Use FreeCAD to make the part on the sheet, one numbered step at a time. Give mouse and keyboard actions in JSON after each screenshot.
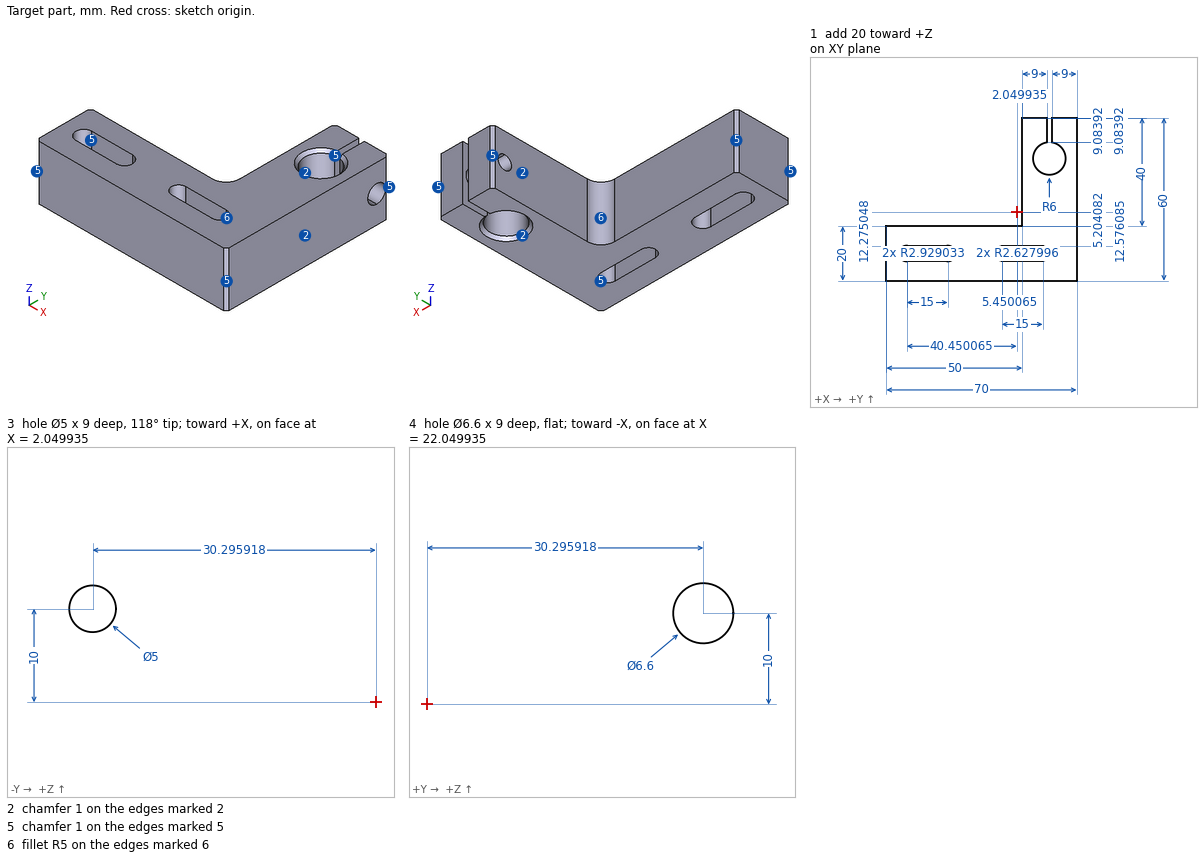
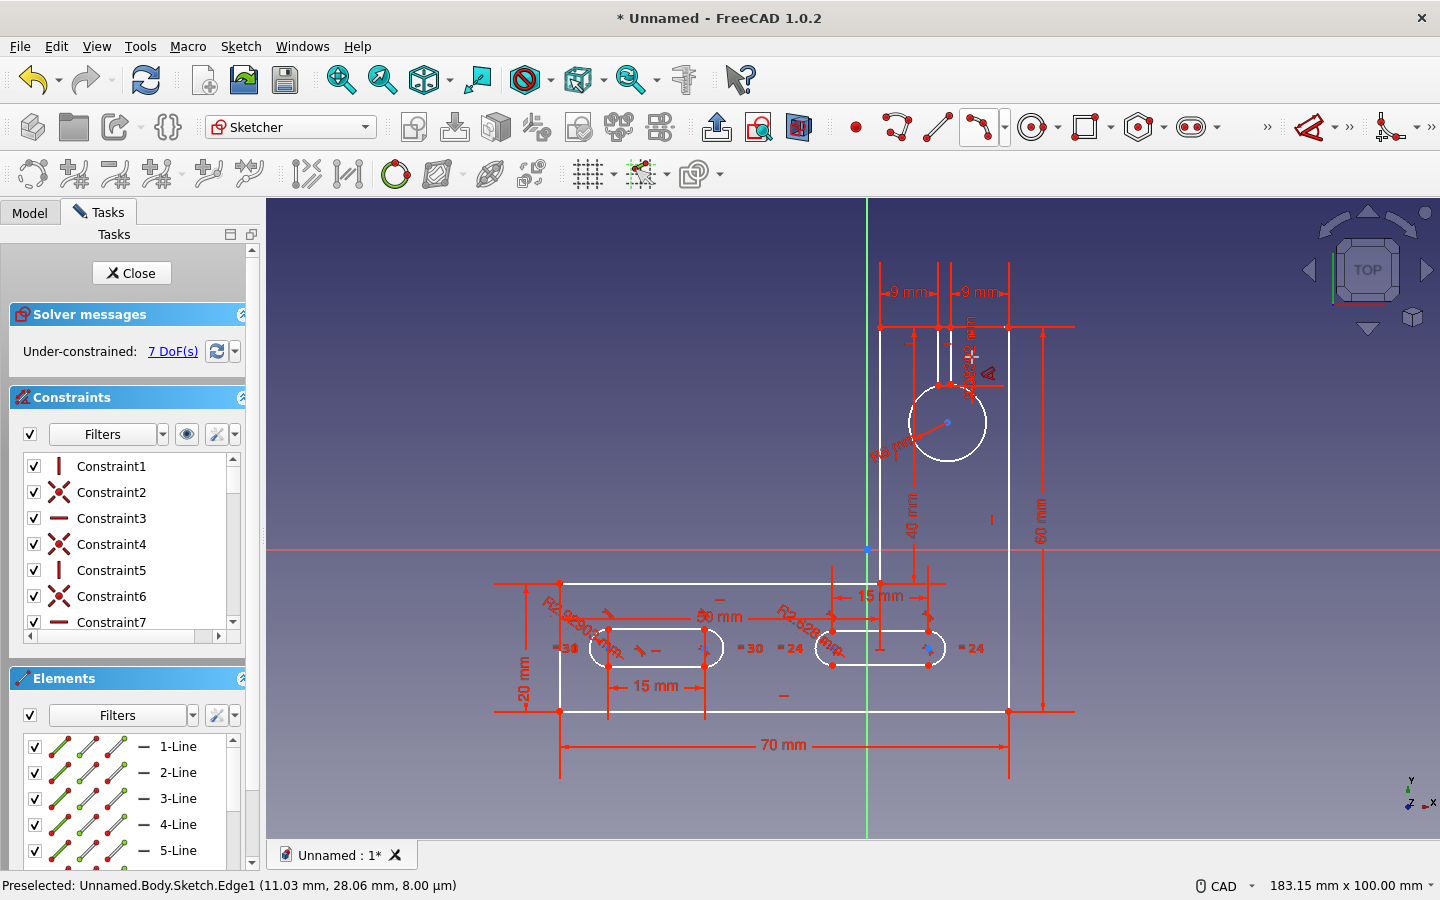
{"action": "left_click", "coordinate": [951, 345]}
{"action": "left_click", "coordinate": [1033, 336]}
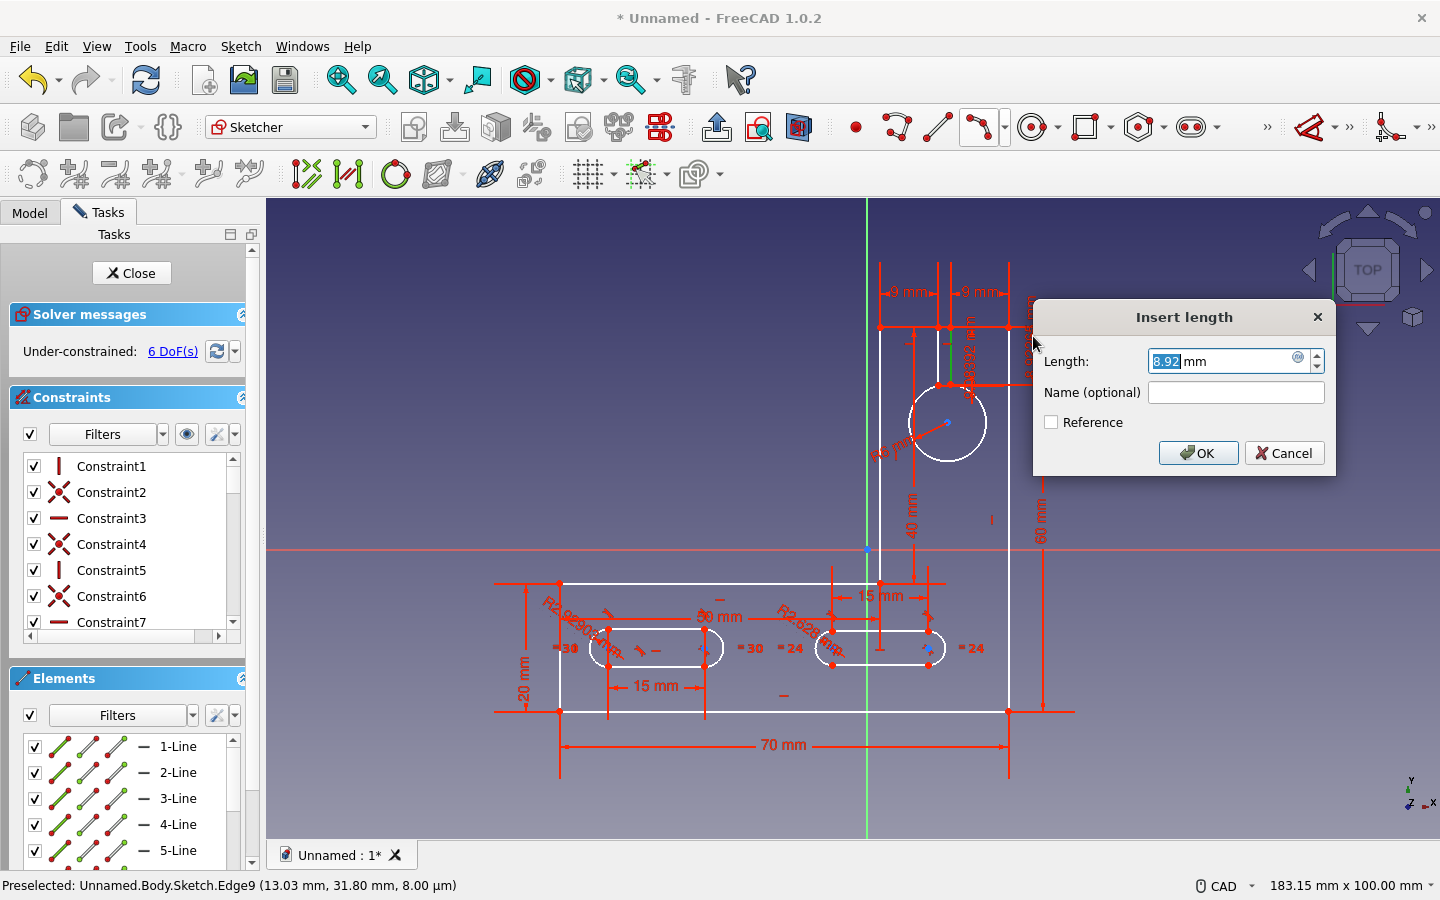
{"action": "type", "text": "9.08392"}
{"action": "key", "text": "Return"}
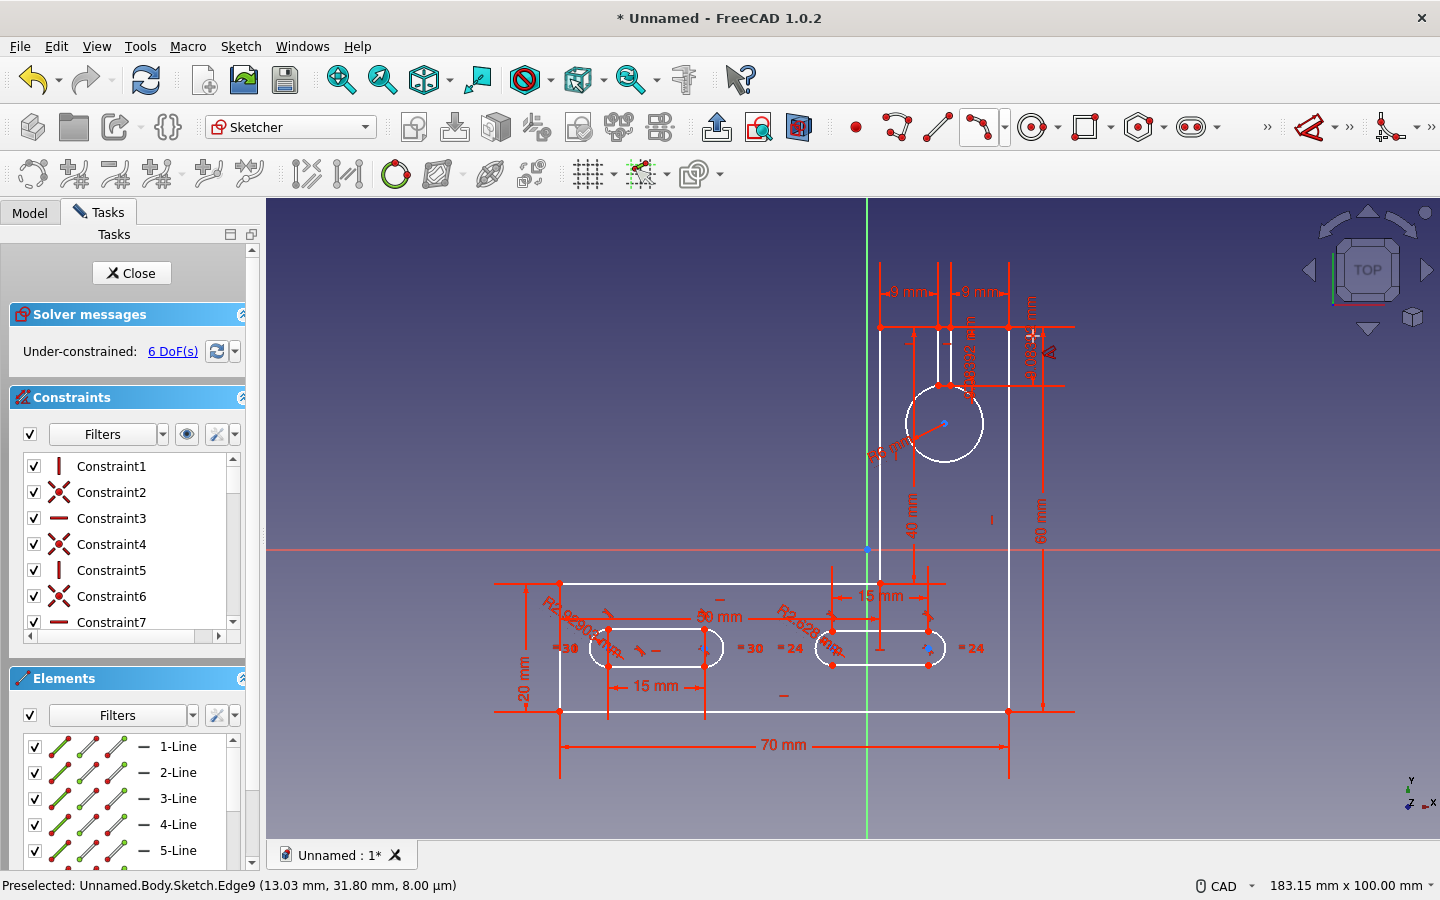
{"action": "scroll", "coordinate": [880, 327], "scroll_direction": "up", "scroll_amount": 6}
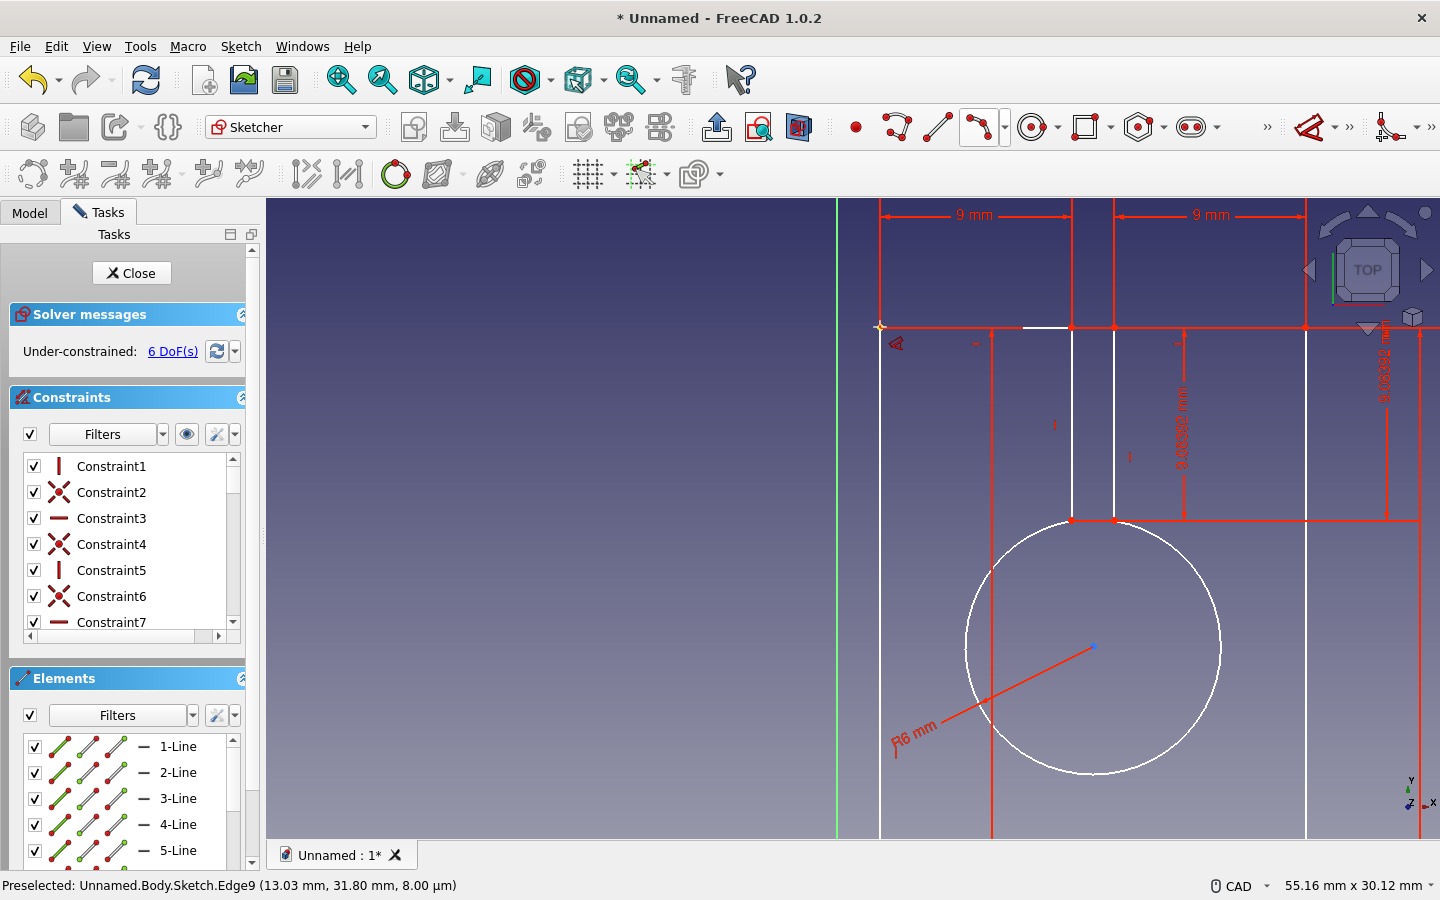
{"action": "left_click", "coordinate": [880, 328]}
{"action": "left_click", "coordinate": [859, 294]}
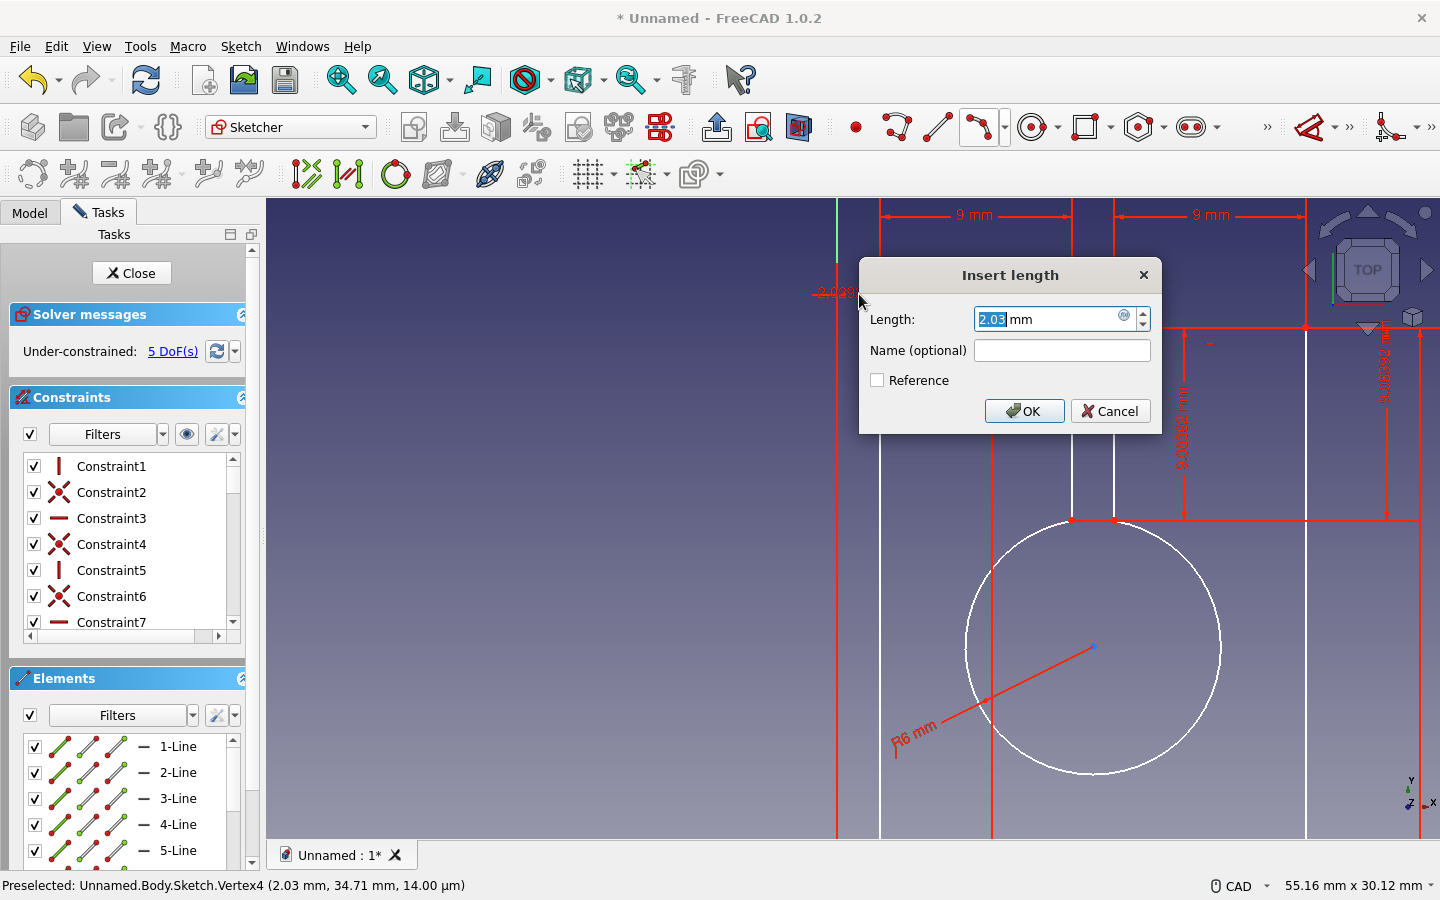
{"action": "type", "text": "2.049935"}
{"action": "key", "text": "Return"}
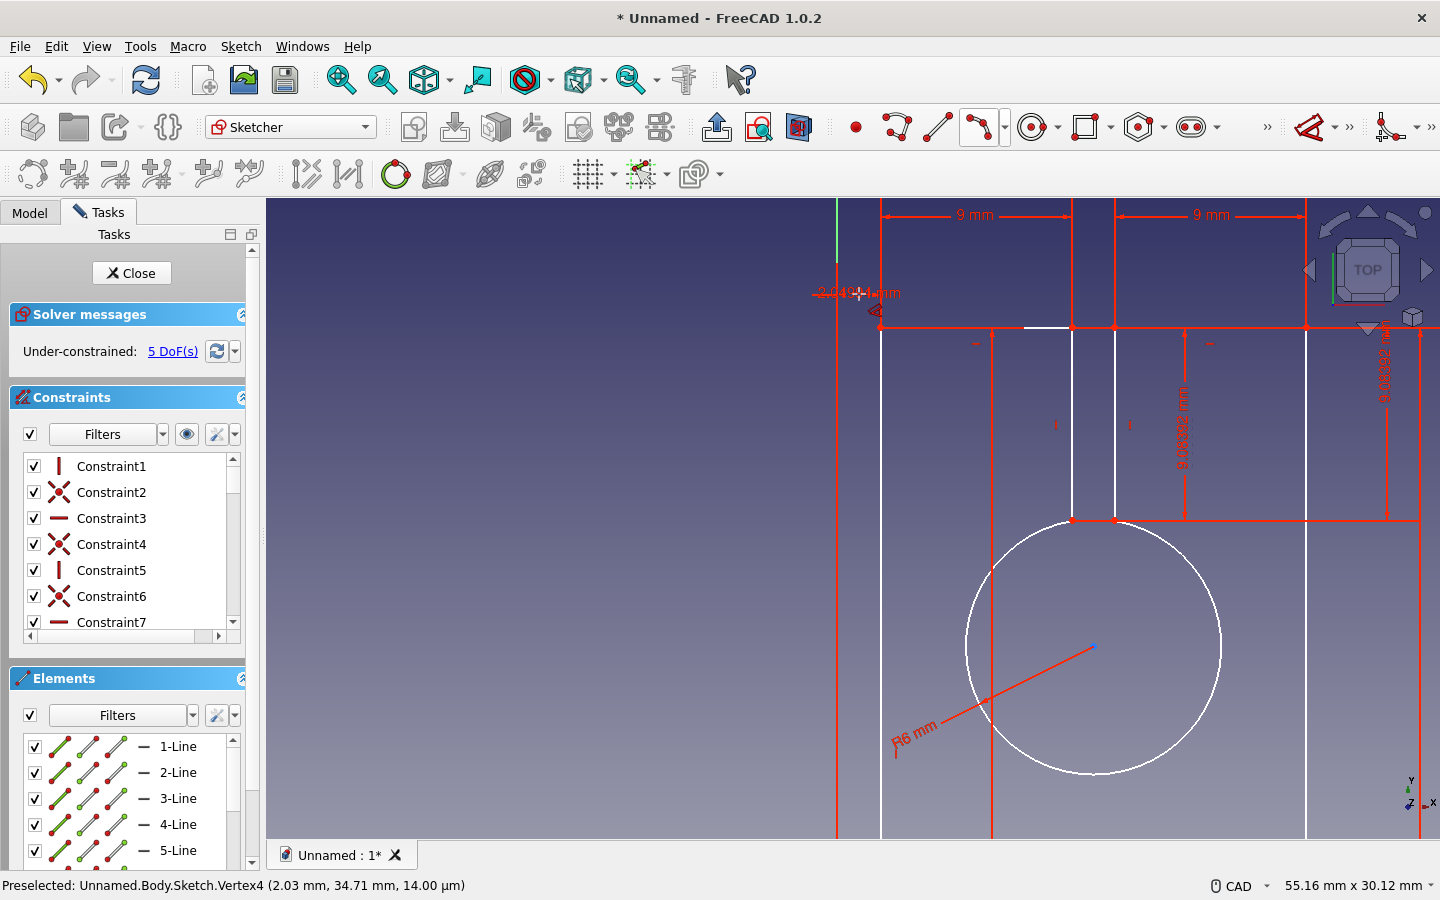
{"action": "scroll", "coordinate": [881, 326], "scroll_direction": "down", "scroll_amount": 6}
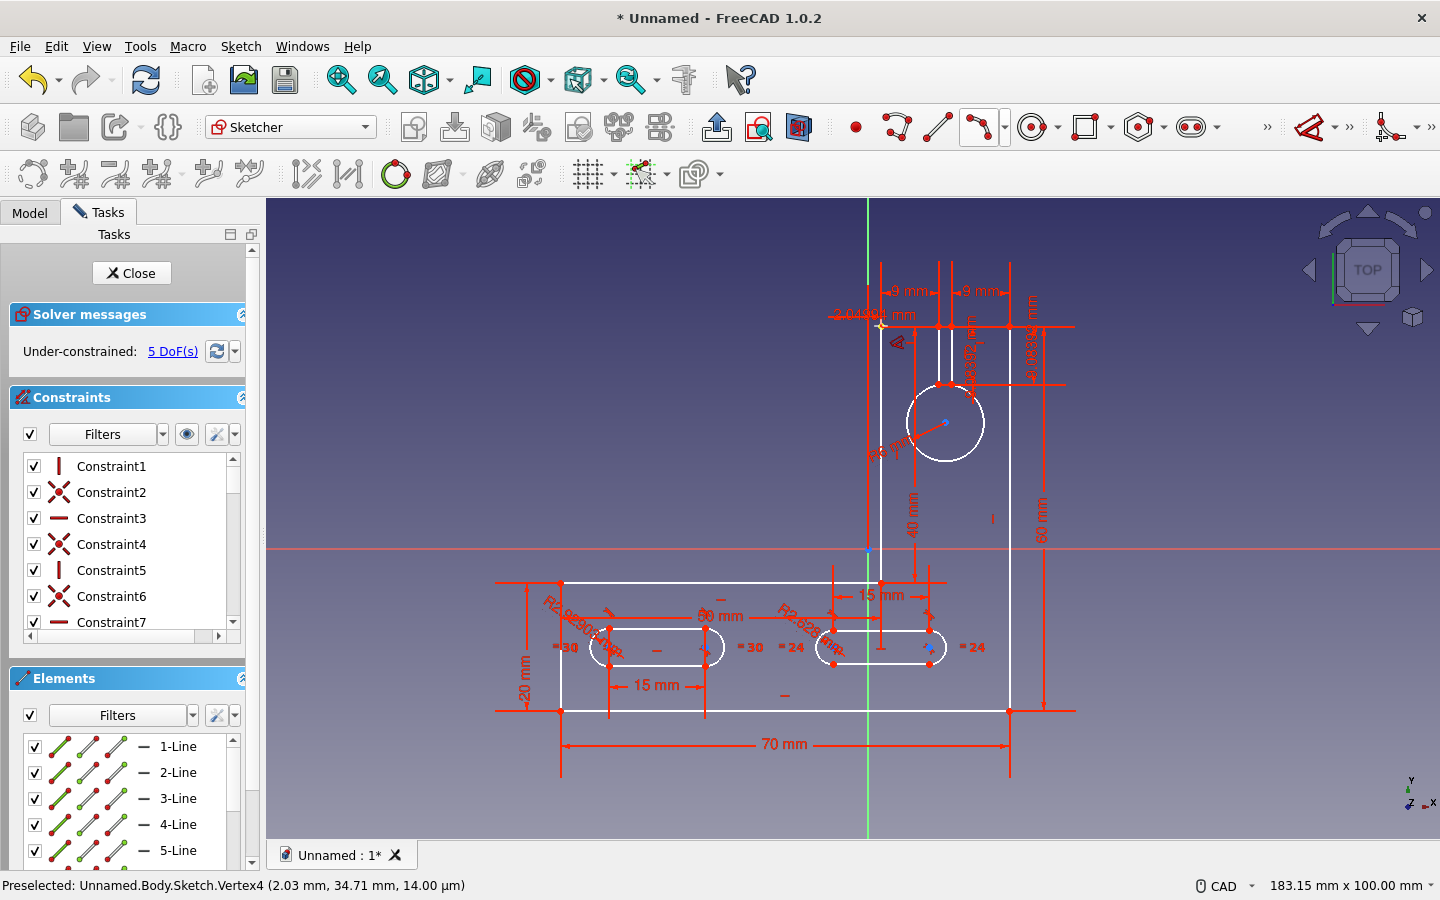
{"action": "left_click", "coordinate": [881, 583]}
{"action": "left_click", "coordinate": [915, 566]}